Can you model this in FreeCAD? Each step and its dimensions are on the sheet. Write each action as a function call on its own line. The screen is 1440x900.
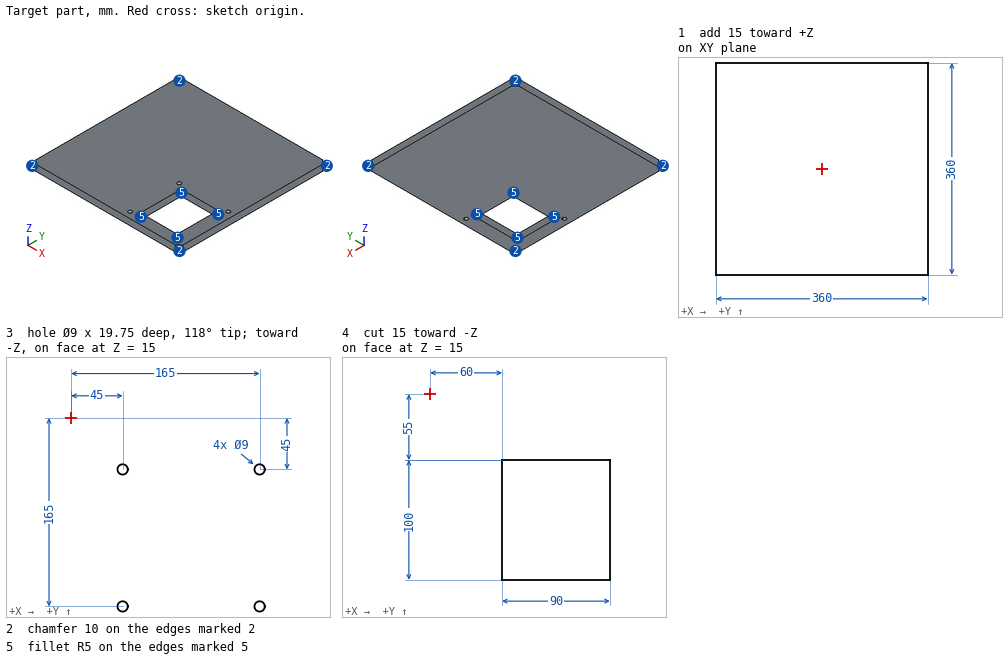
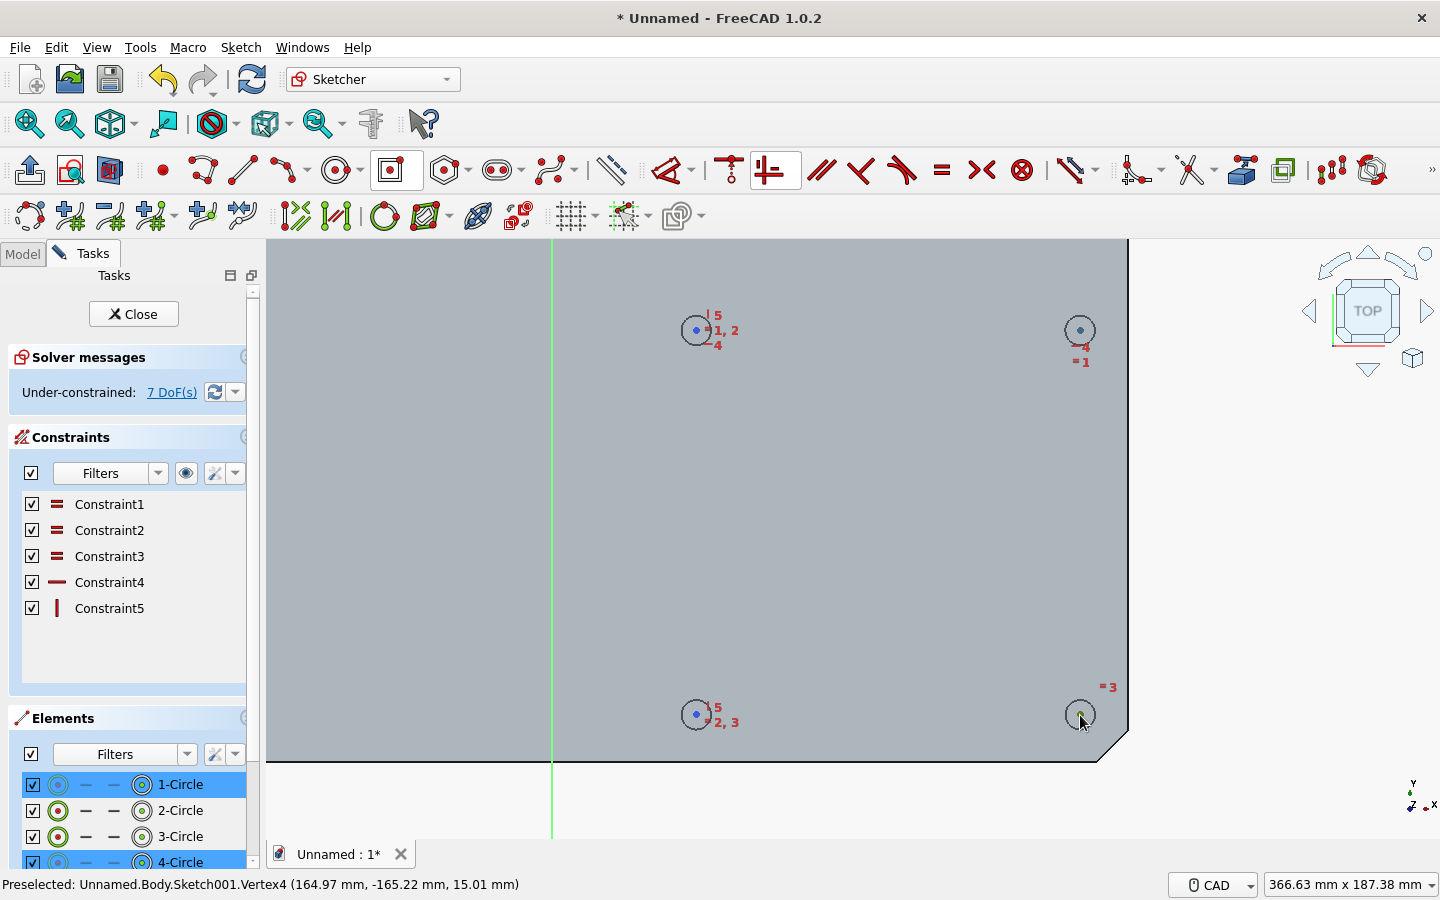
key(v)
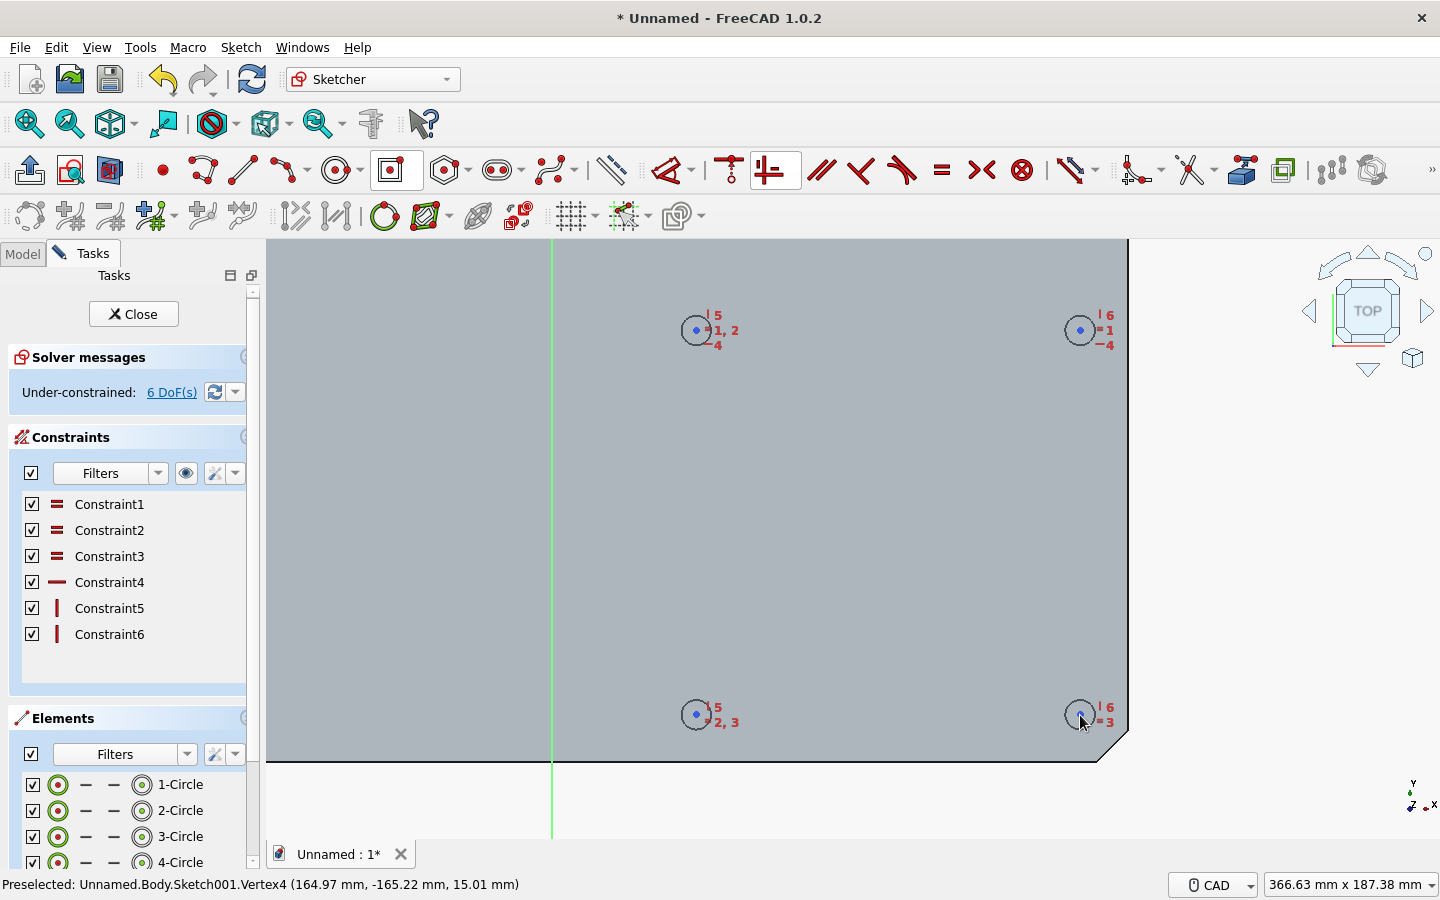
click(696, 715)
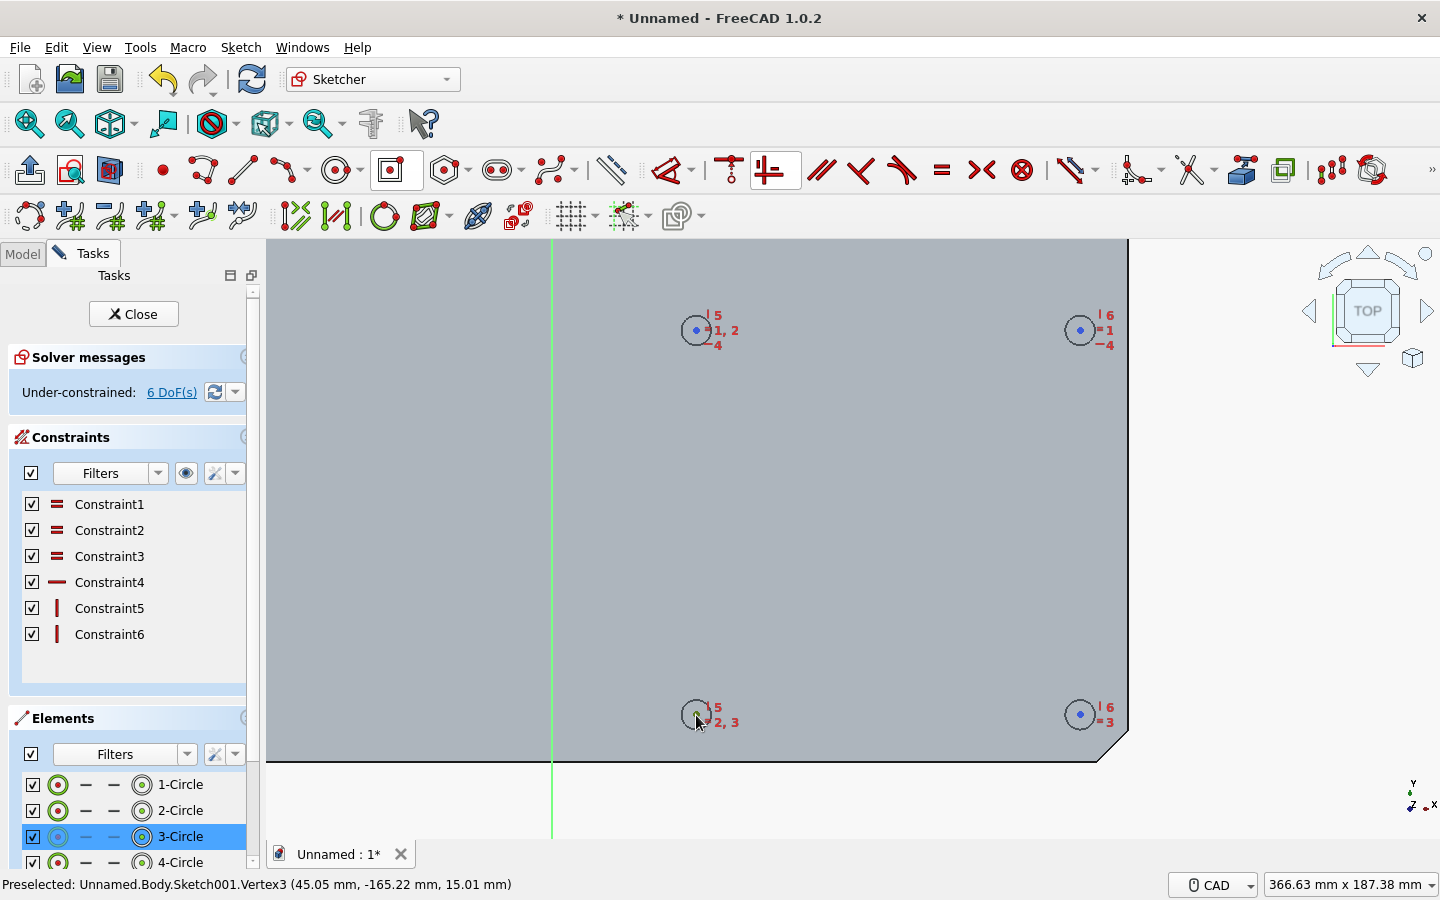
click(1080, 715)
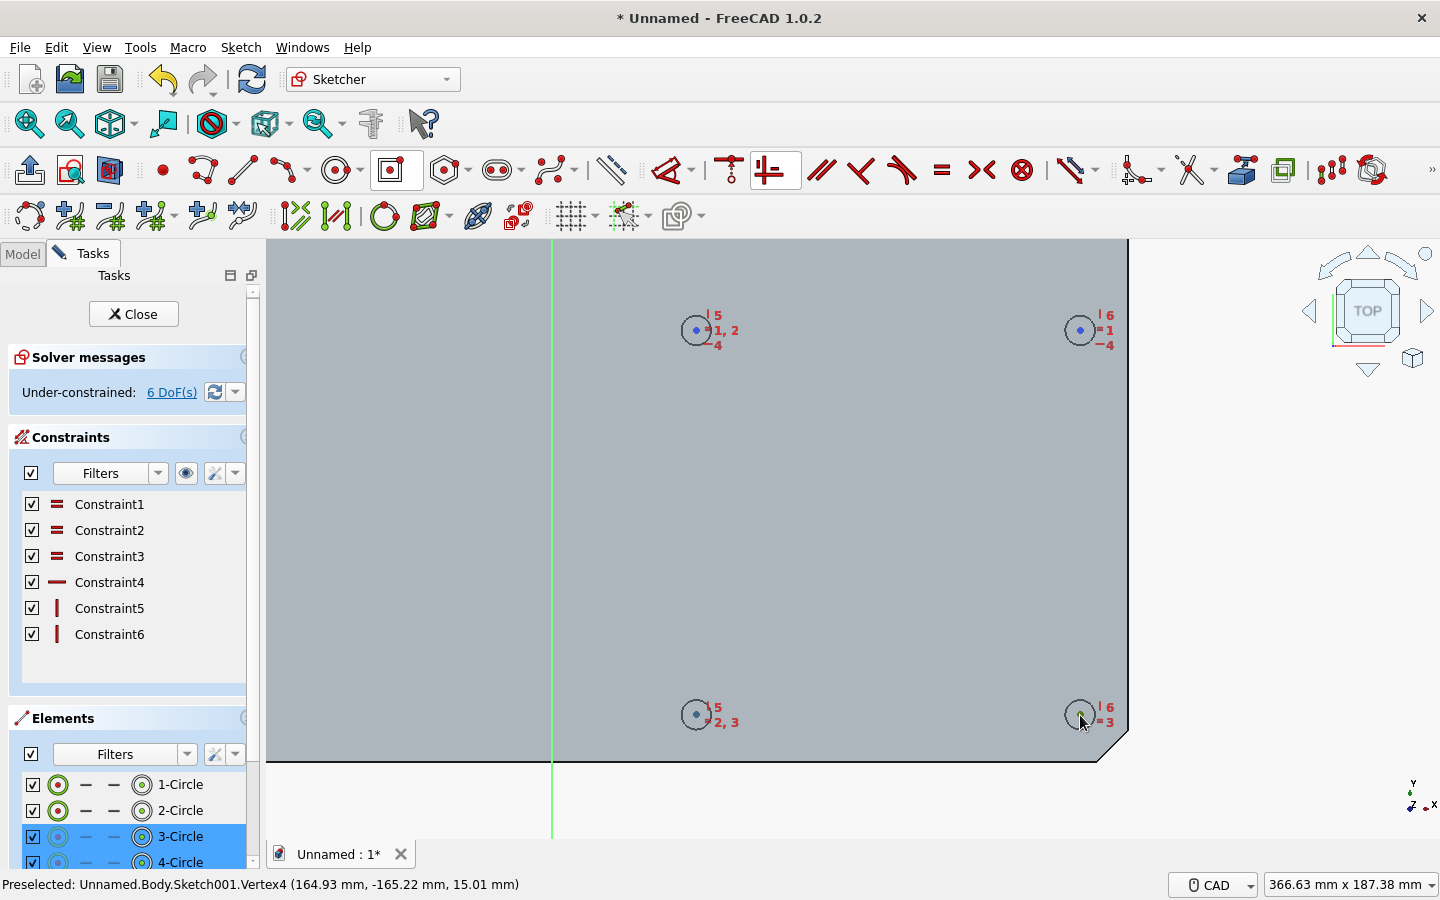
key(h)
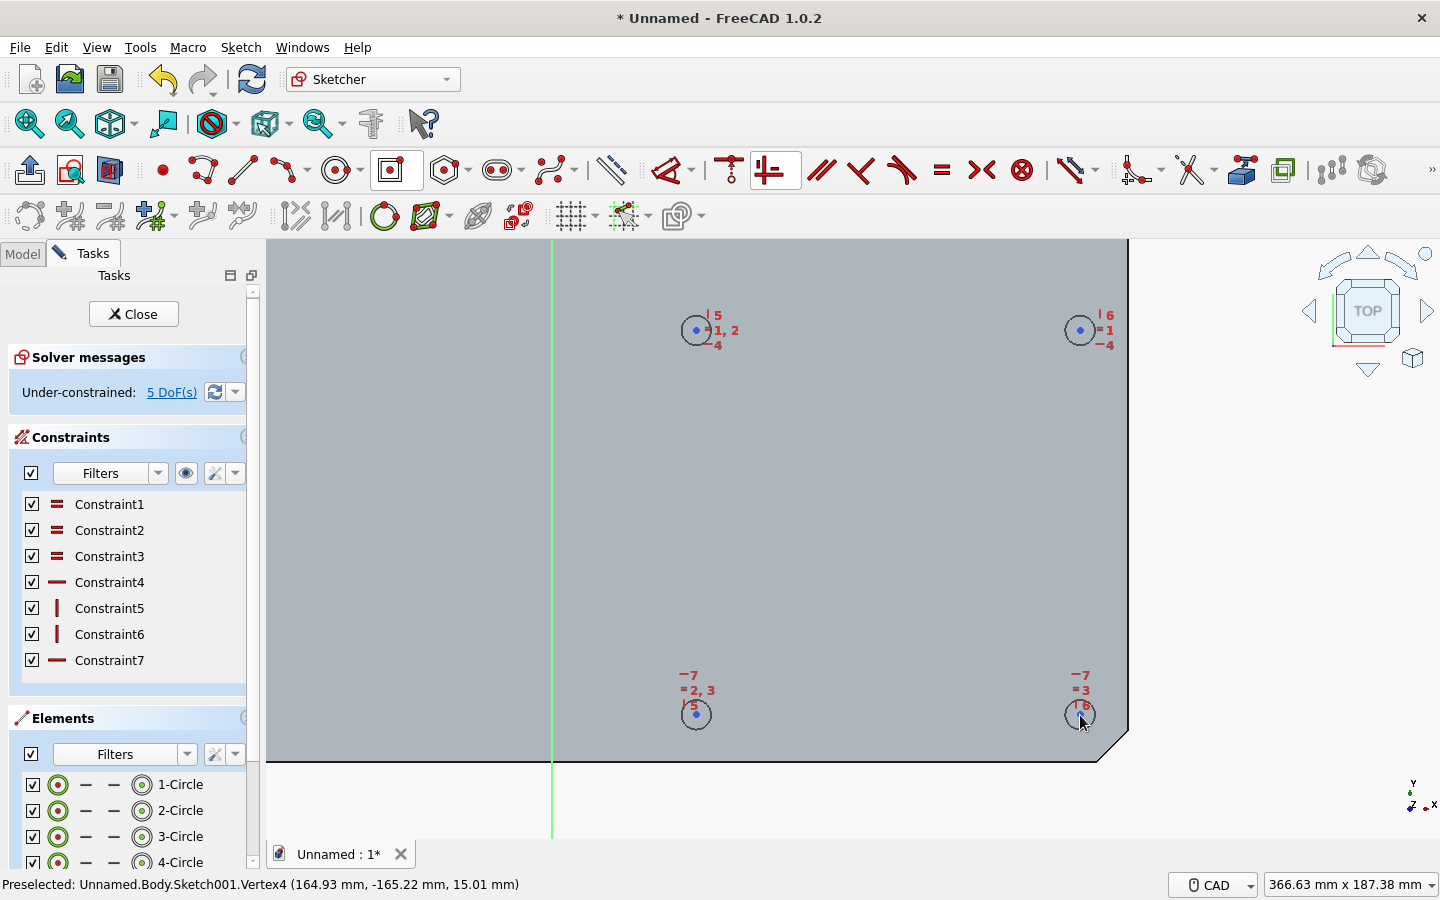
click(666, 170)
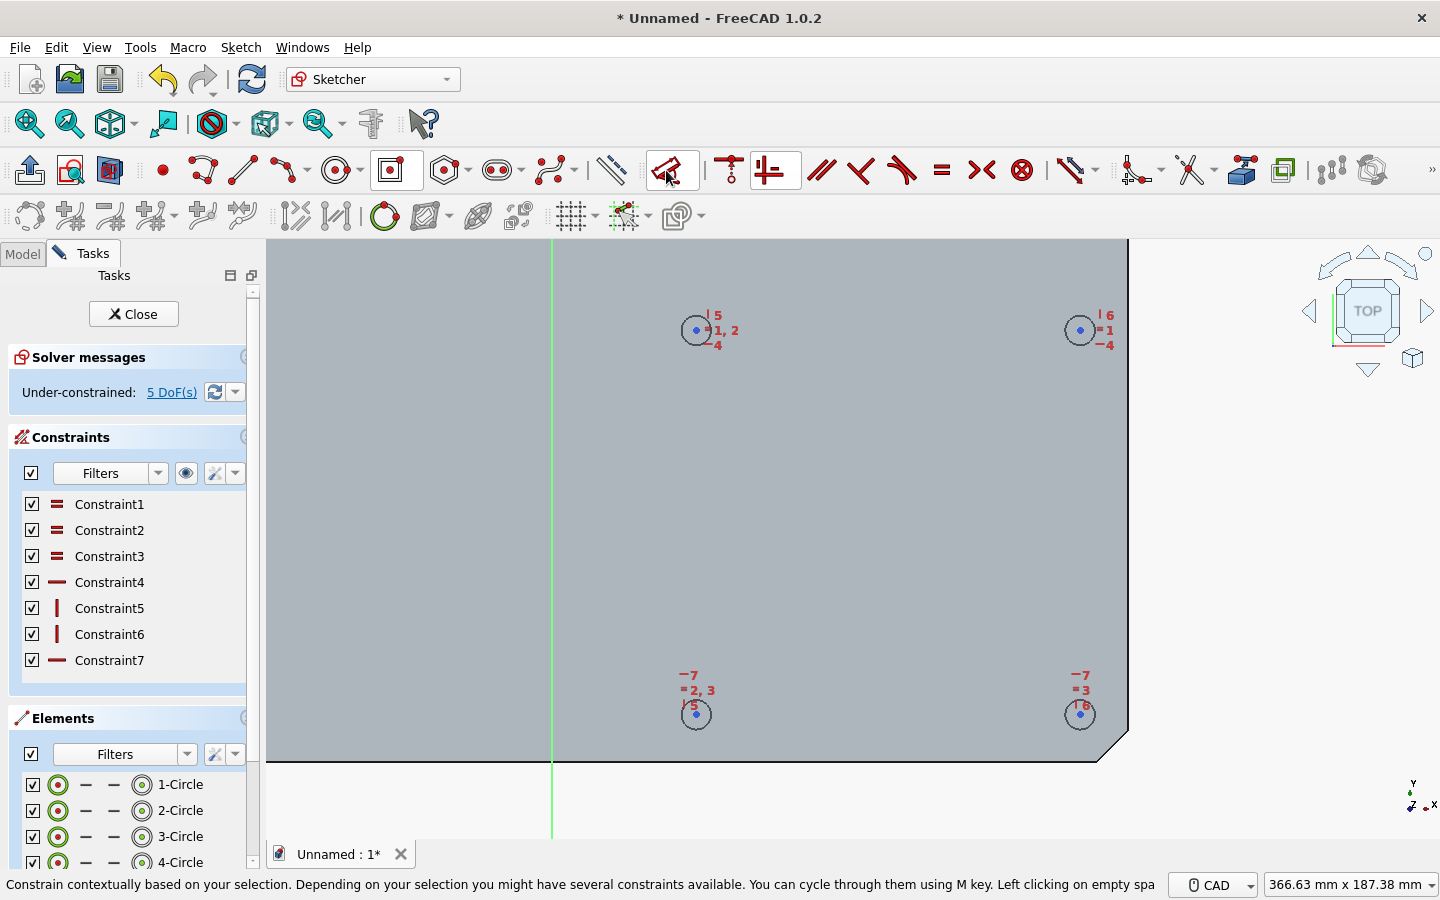
scroll(1091, 320, up, 2)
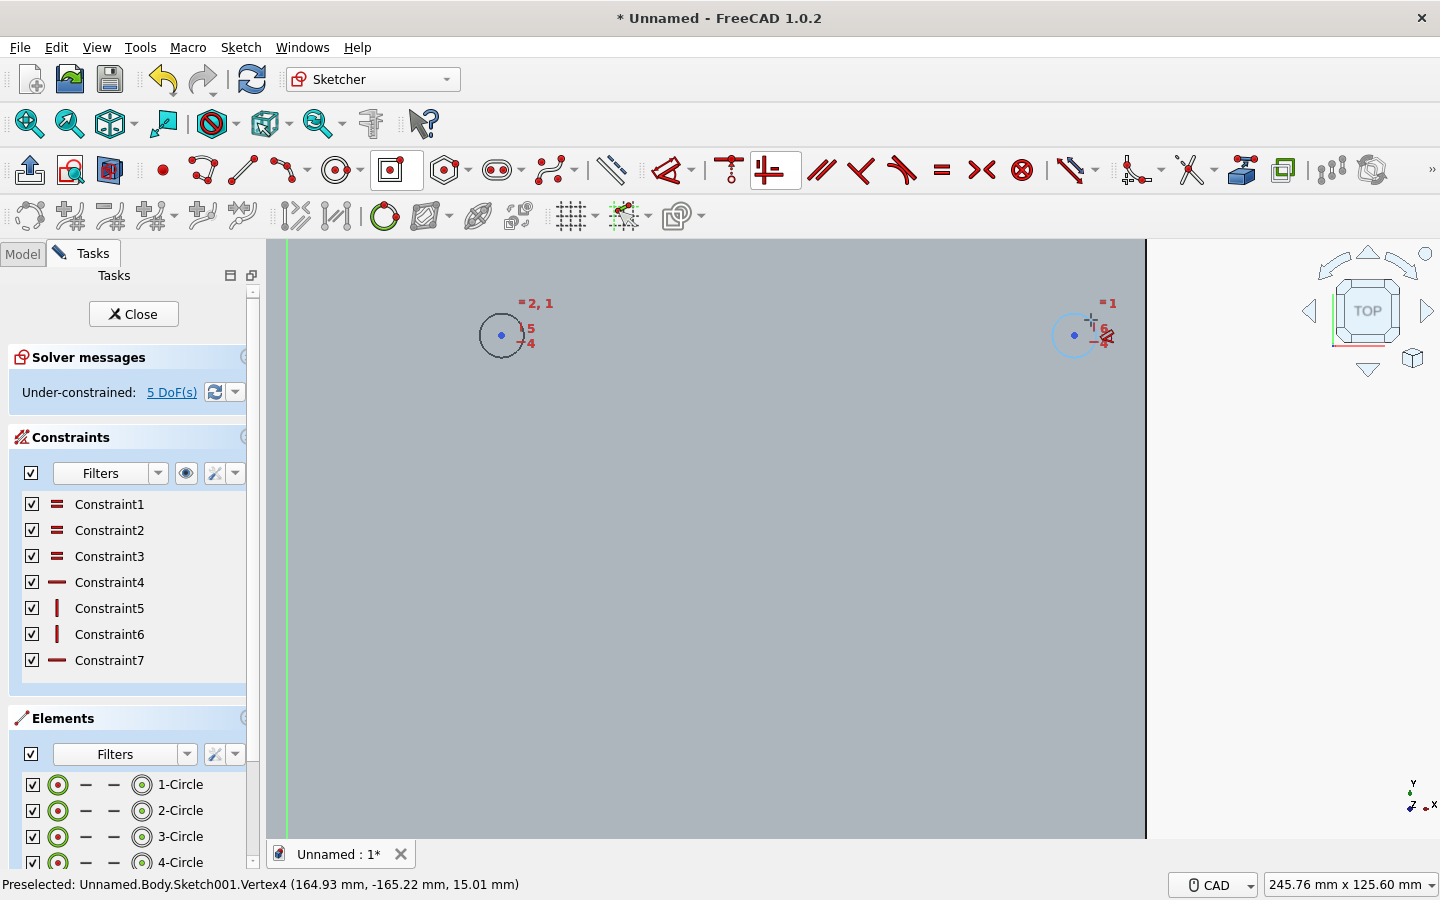
click(1090, 320)
click(1113, 297)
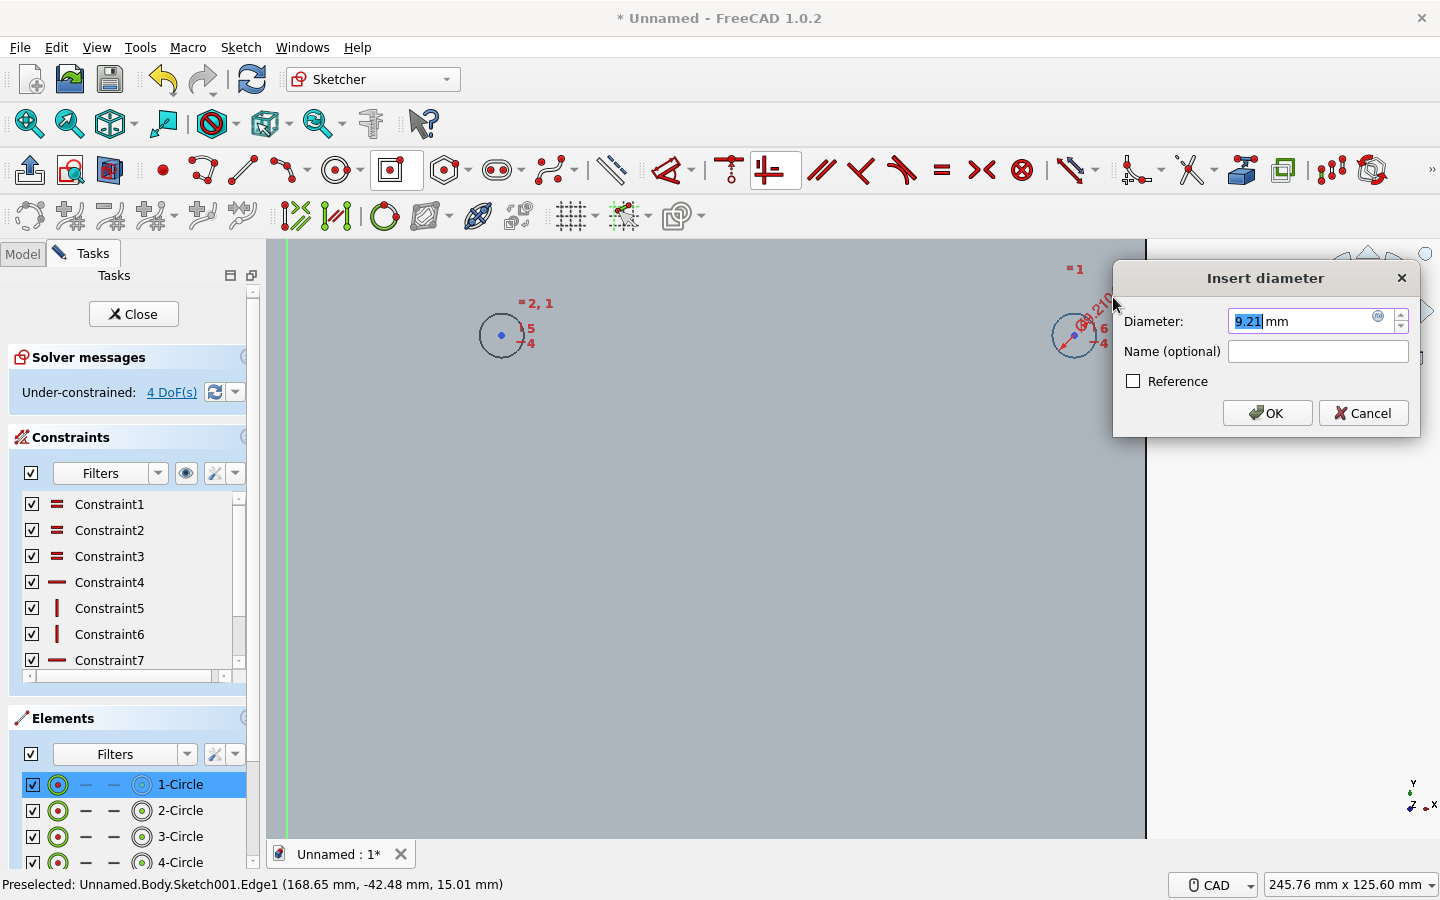
text(9)
key(Return)